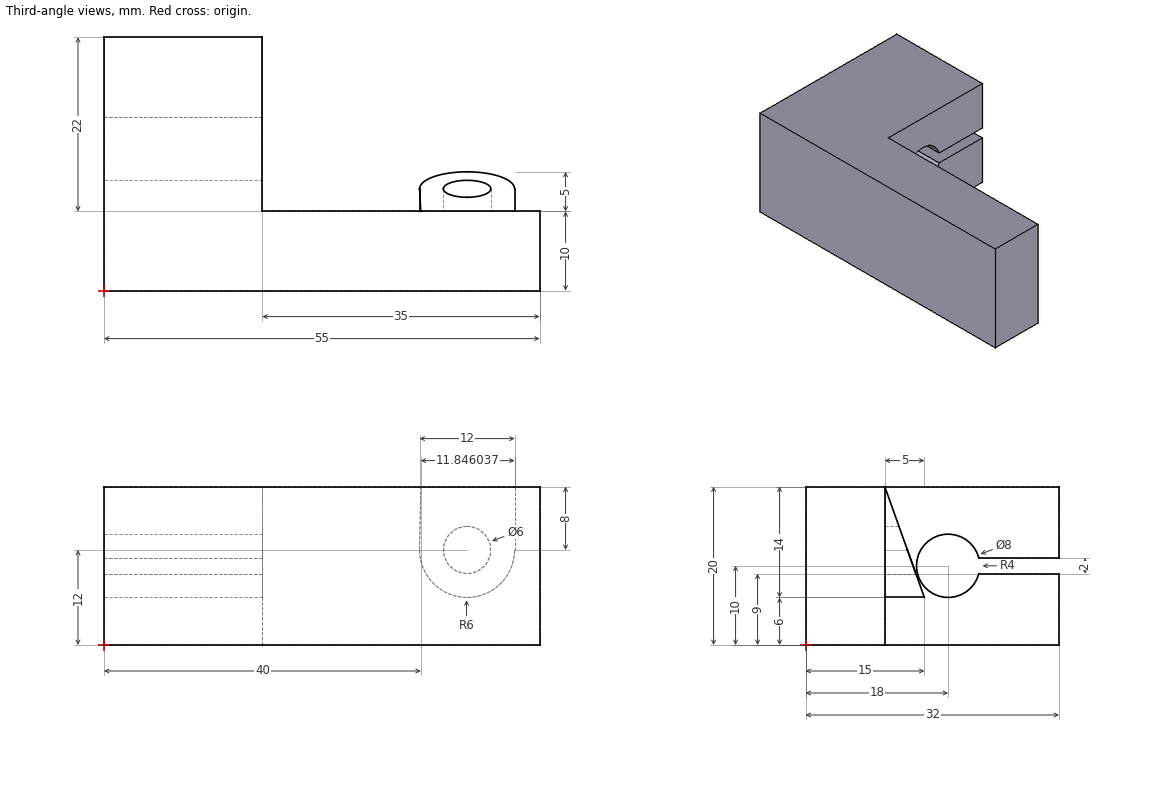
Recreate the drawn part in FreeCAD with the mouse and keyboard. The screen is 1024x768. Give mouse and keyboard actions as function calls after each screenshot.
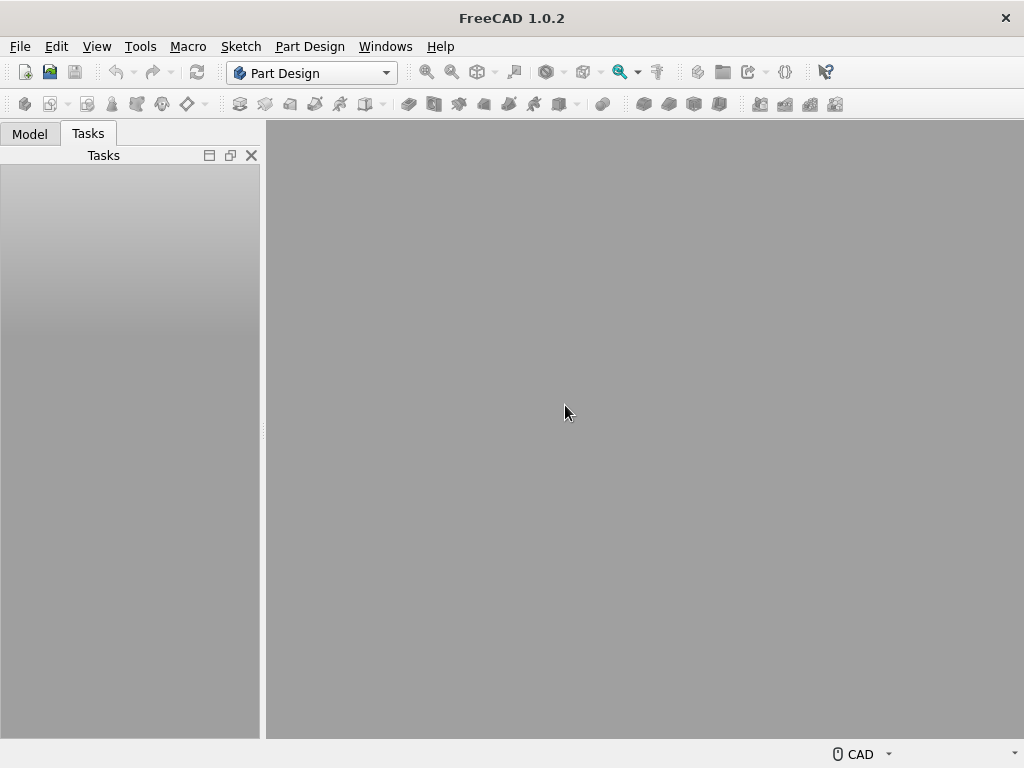
key(ctrl+n)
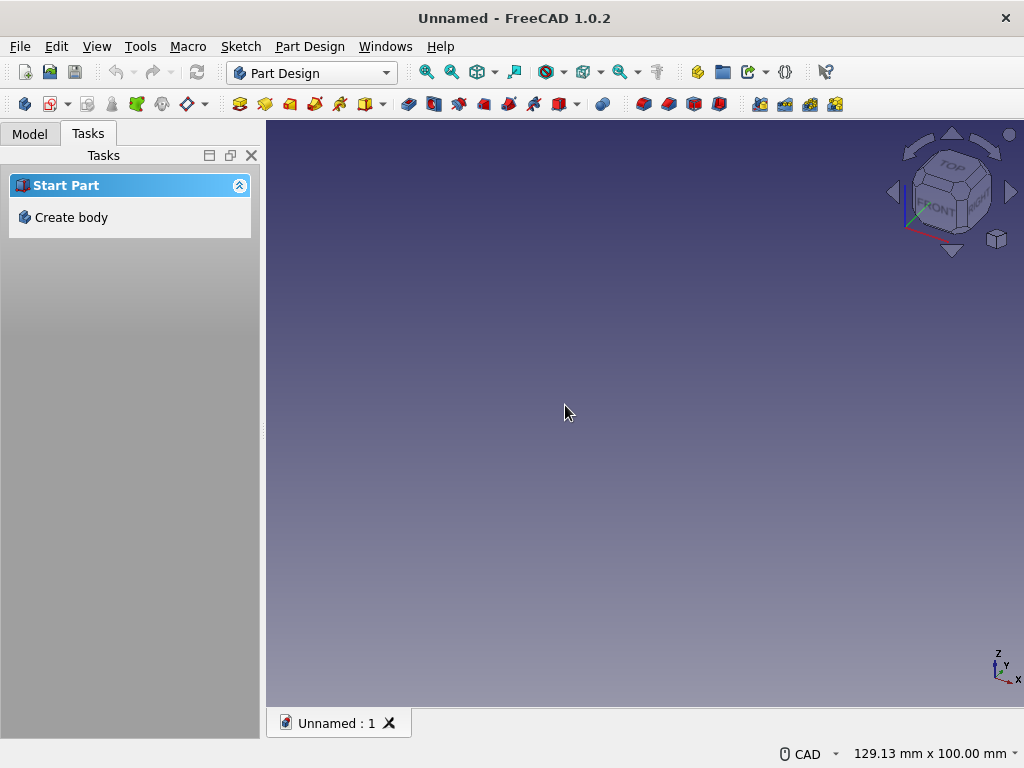
click(50, 104)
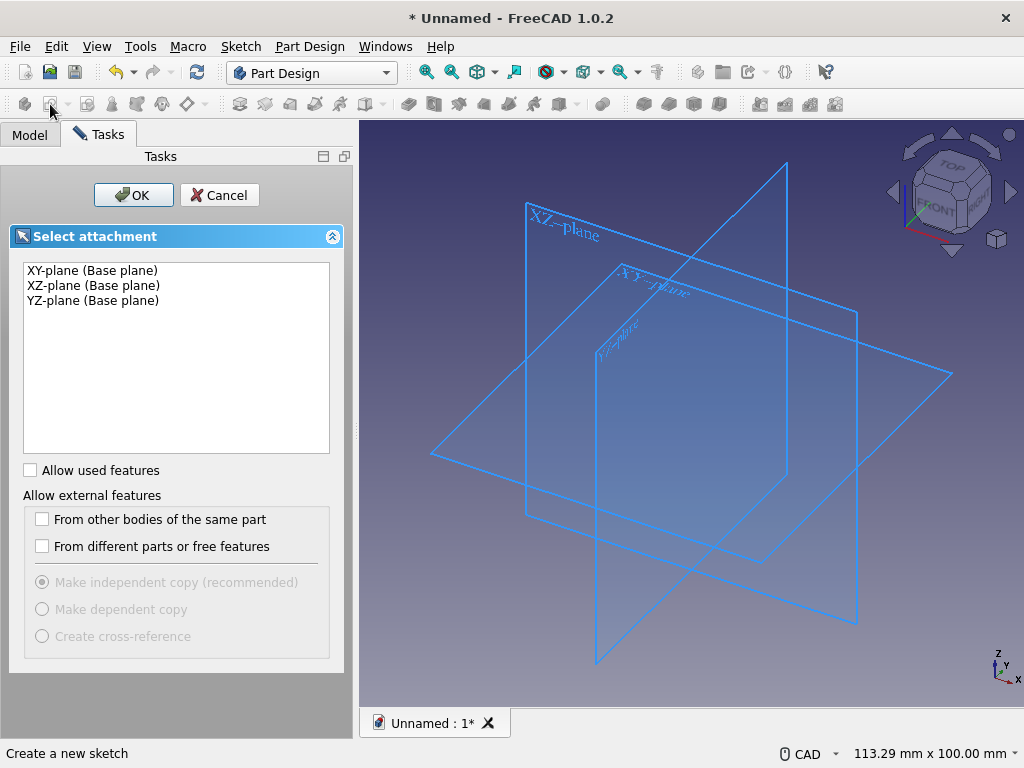
click(84, 270)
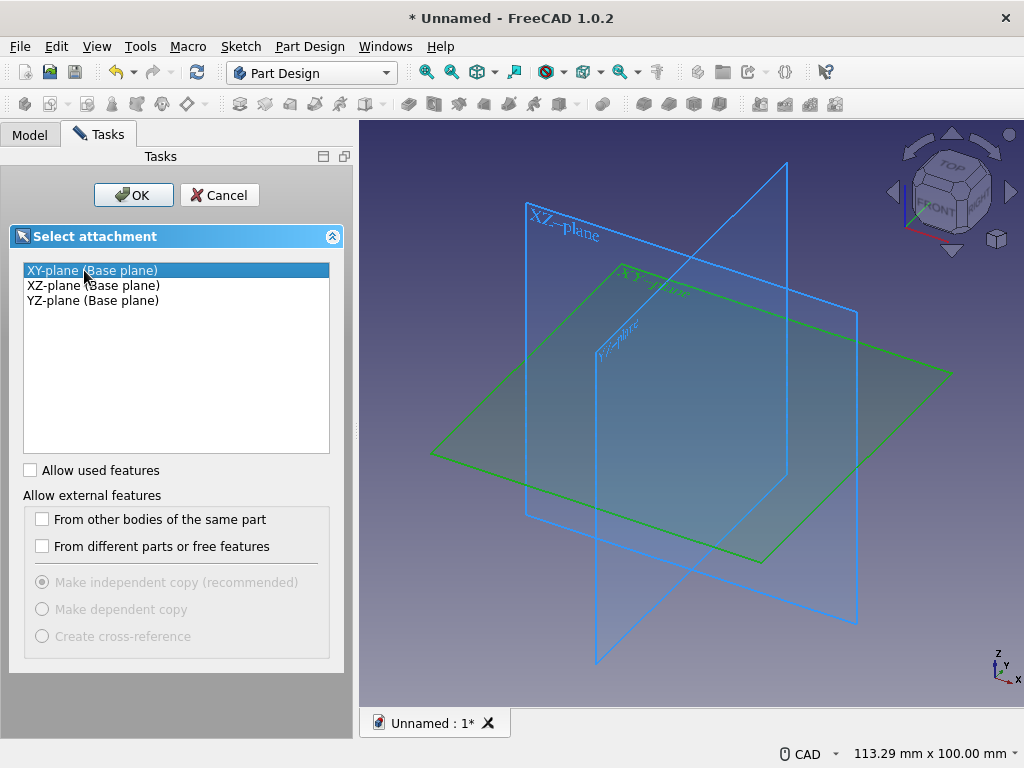
click(134, 195)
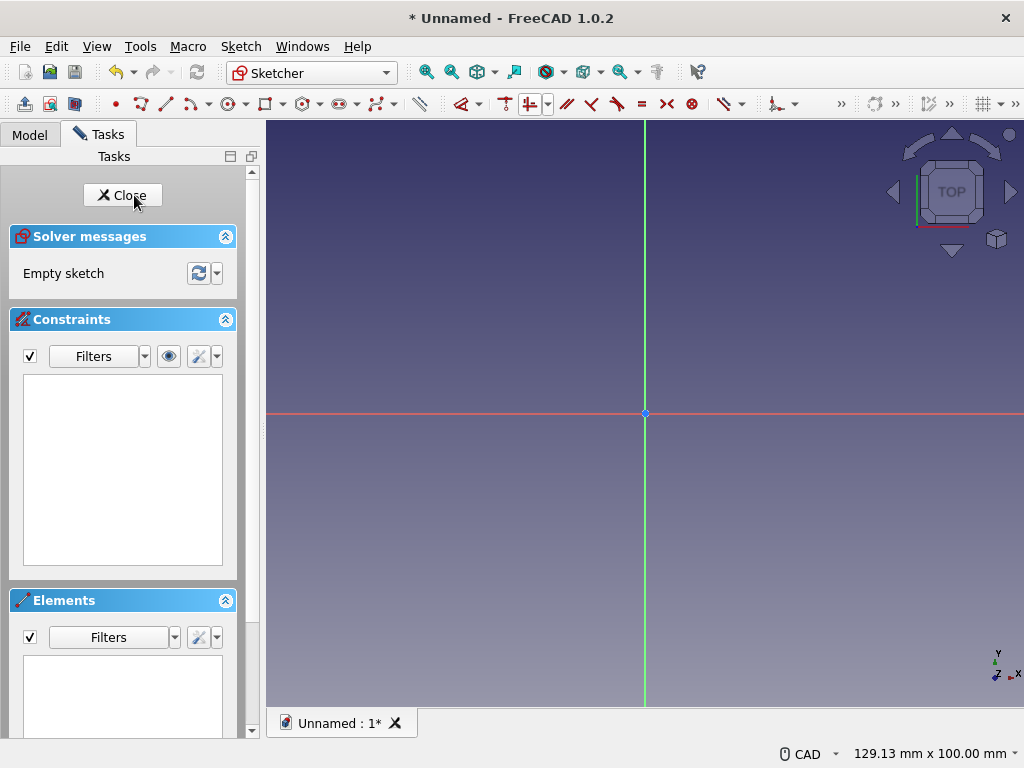
scroll(294, 604, down, 2)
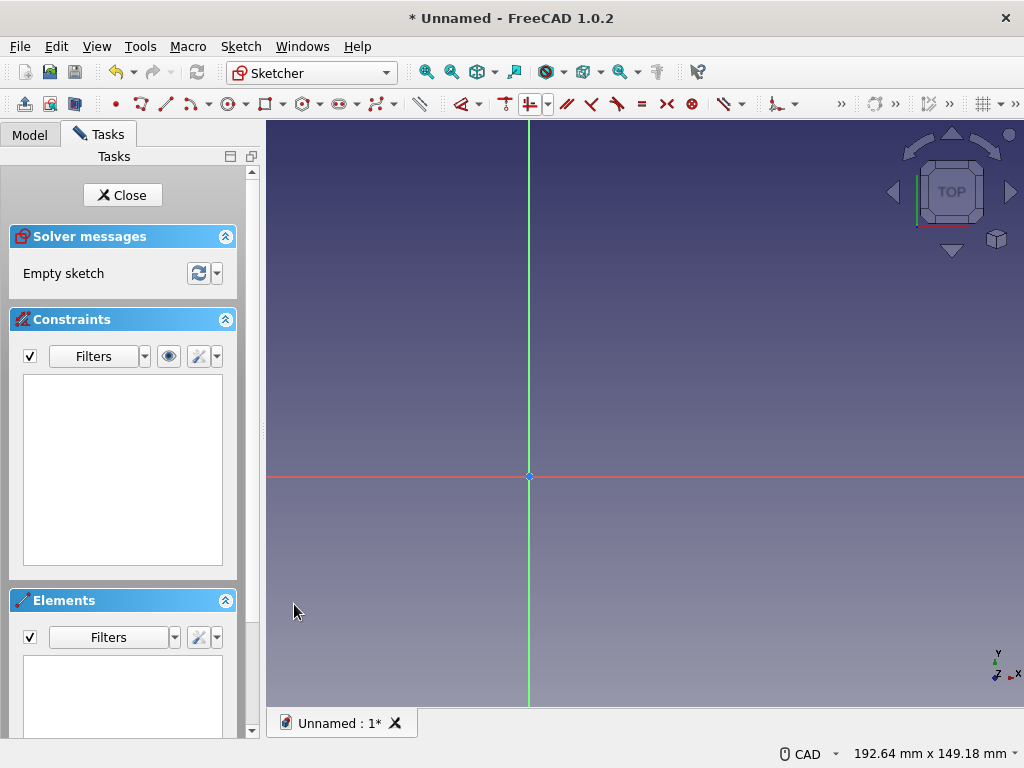
scroll(712, 414, up, 3)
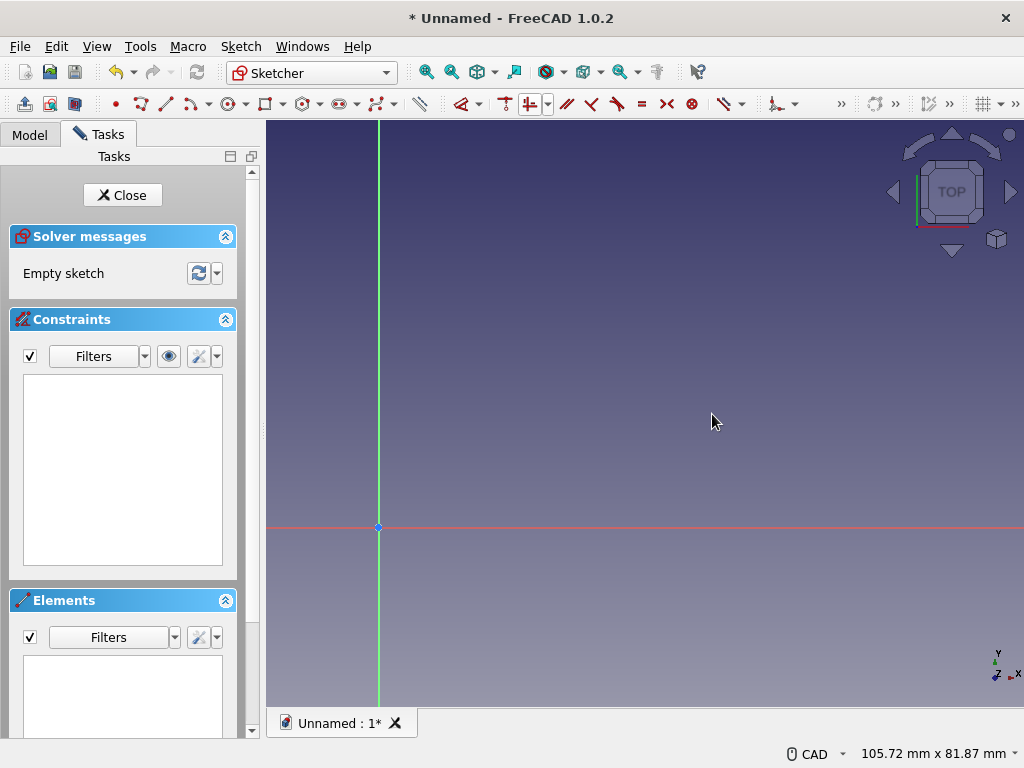
click(141, 104)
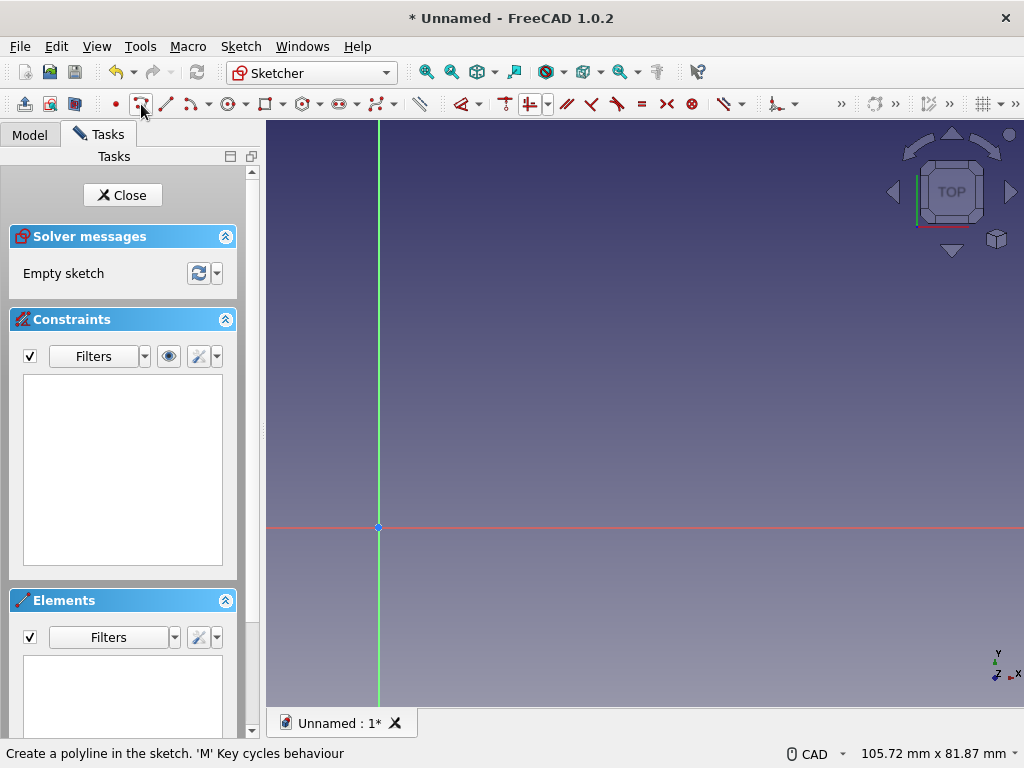
click(379, 528)
click(773, 519)
click(773, 456)
click(522, 456)
click(522, 298)
click(388, 298)
click(379, 528)
key(Escape)
key(Escape)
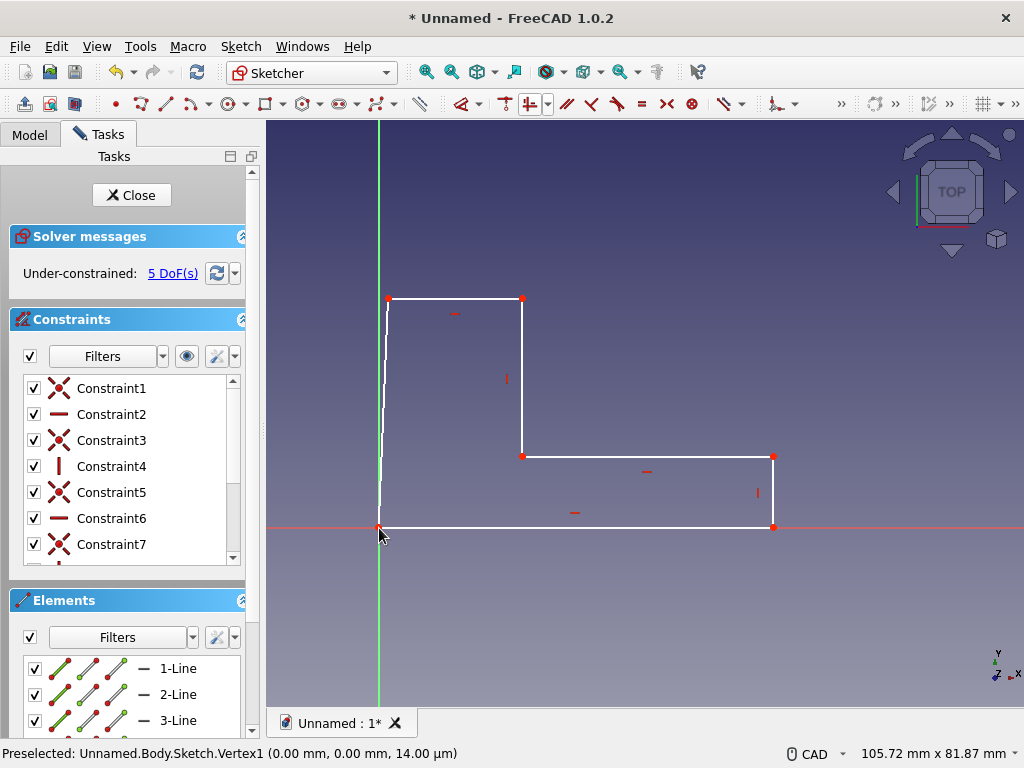
click(381, 459)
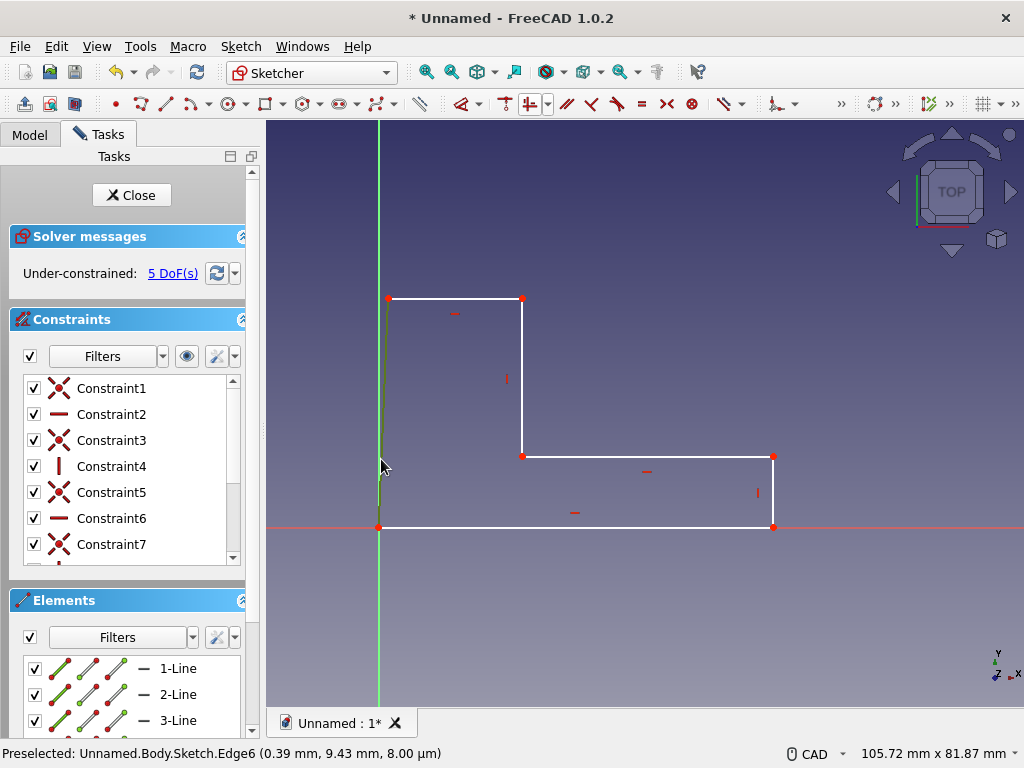
key(v)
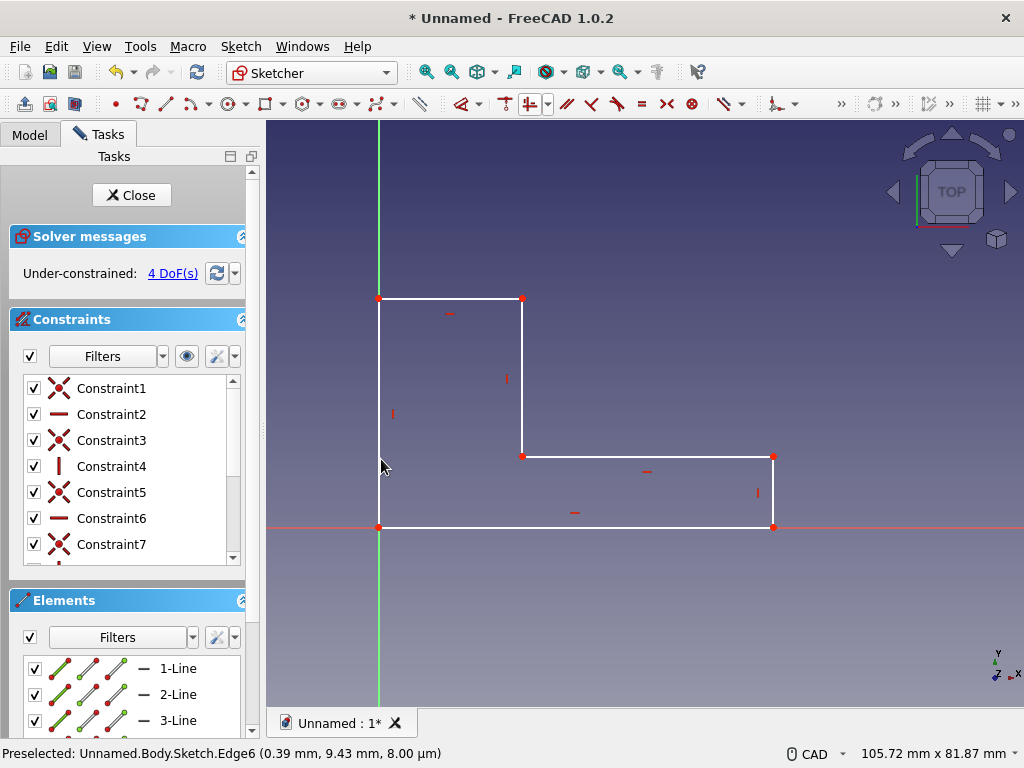
click(460, 104)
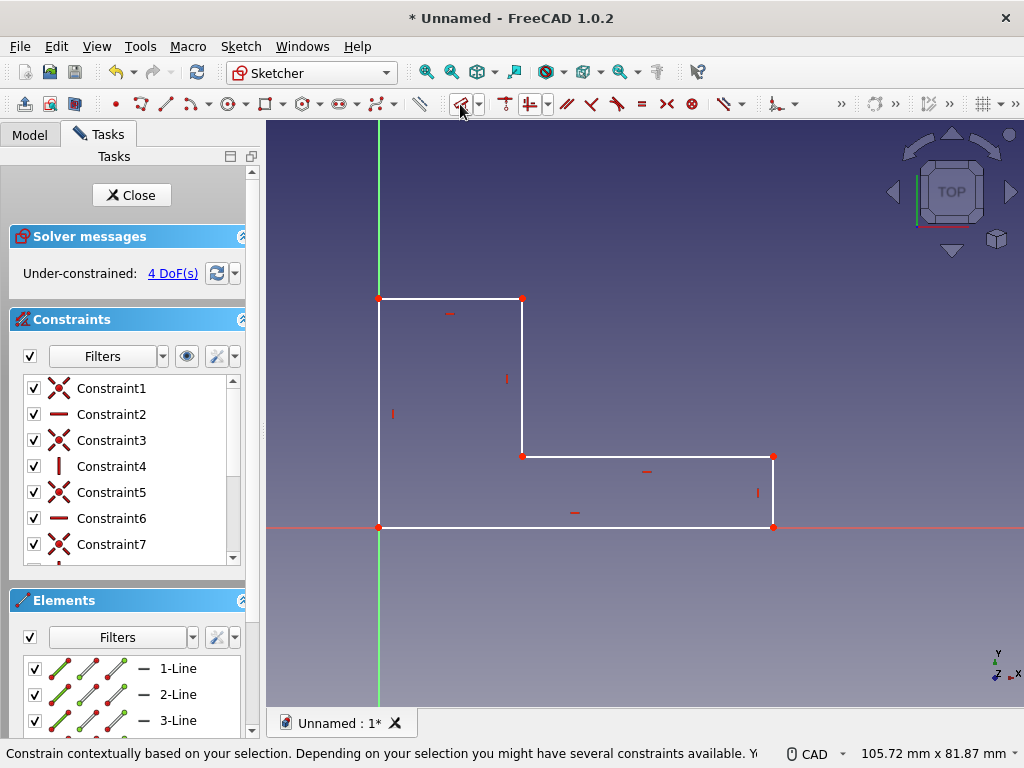
click(497, 528)
click(576, 562)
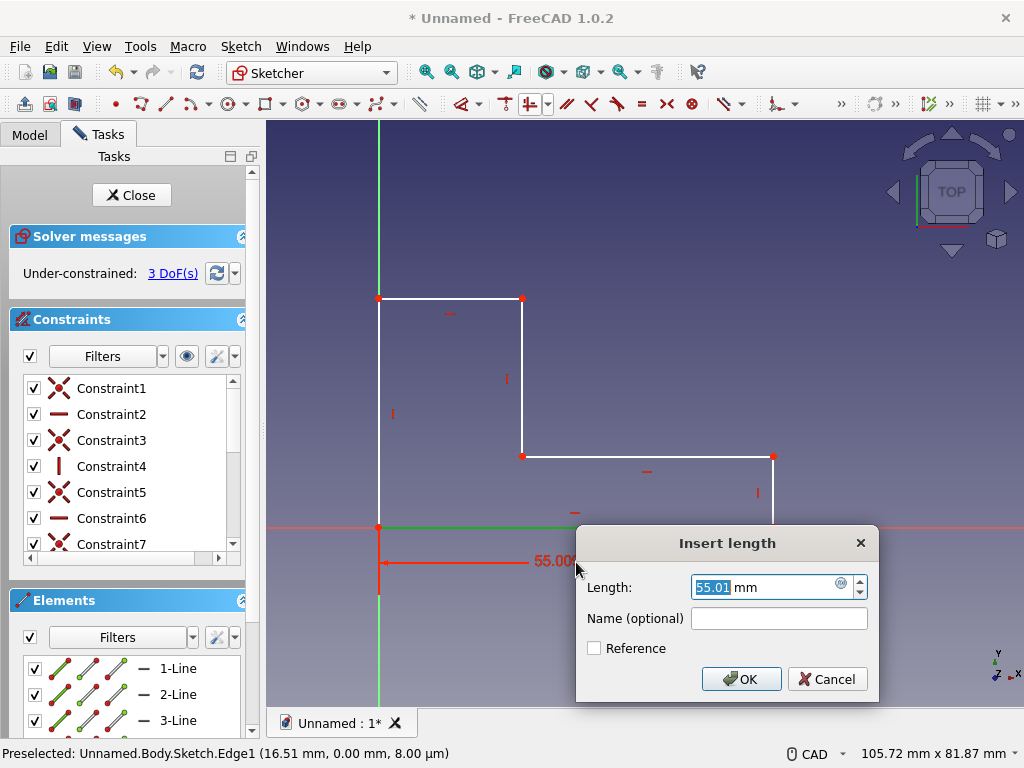
text(55)
key(Return)